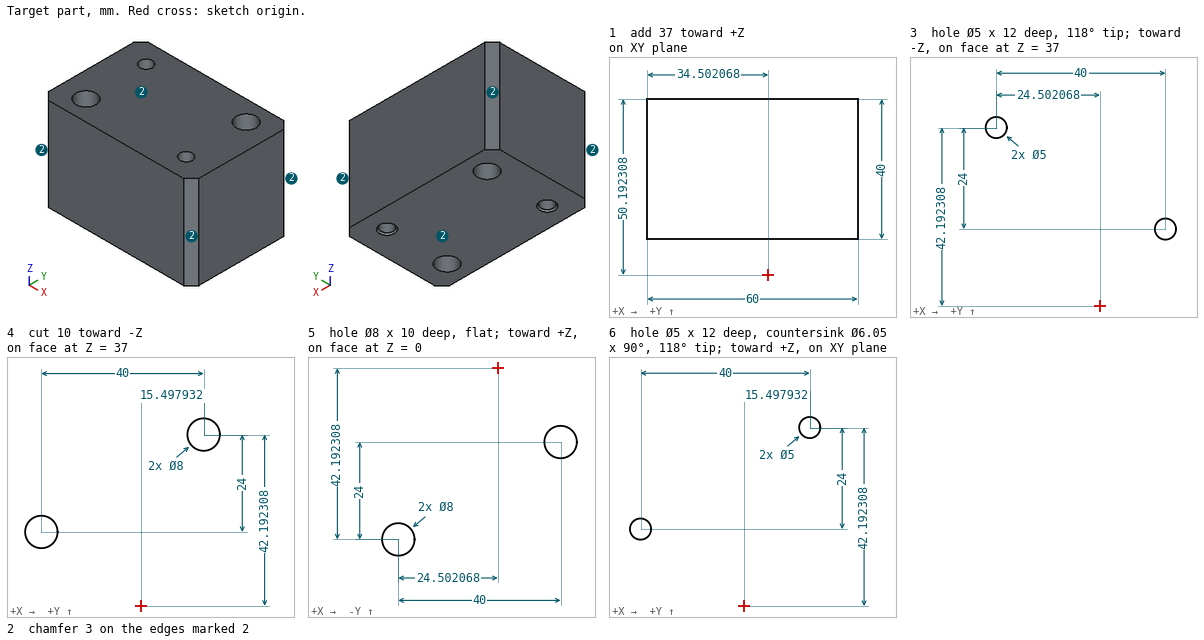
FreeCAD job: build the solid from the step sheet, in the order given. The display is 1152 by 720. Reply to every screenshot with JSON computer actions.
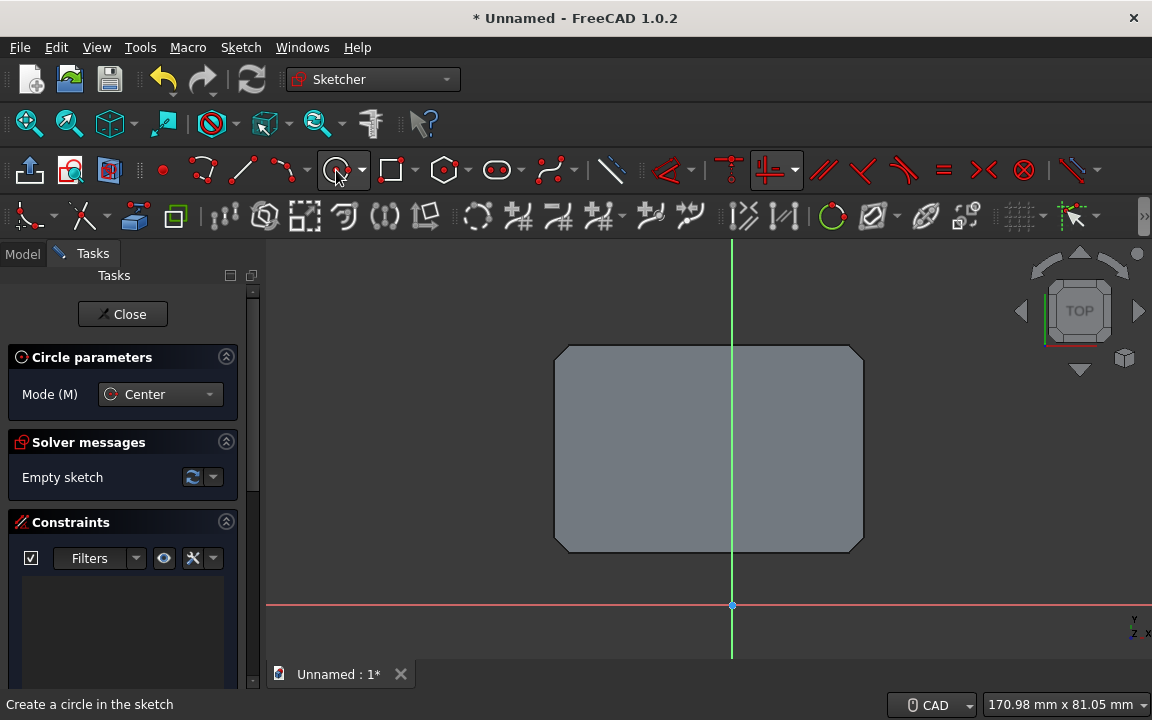
{"action": "scroll", "coordinate": [605, 387], "scroll_direction": "up", "scroll_amount": 3}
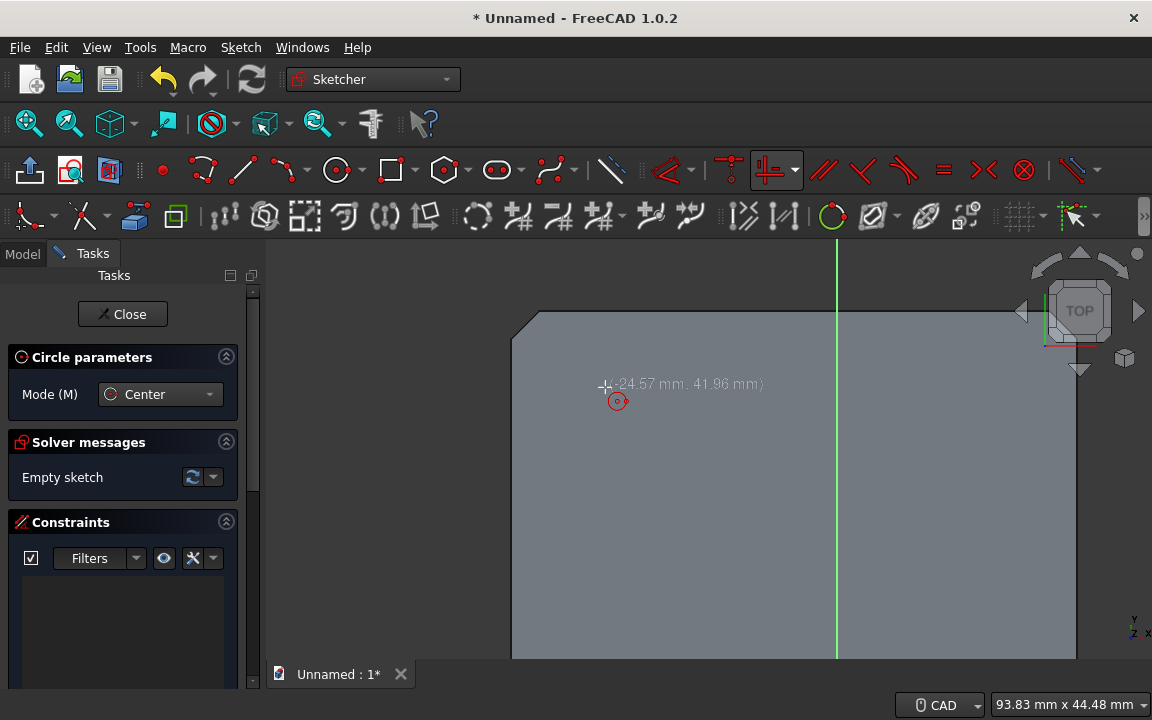
{"action": "left_click", "coordinate": [605, 386]}
{"action": "mouse_move", "coordinate": [622, 370]}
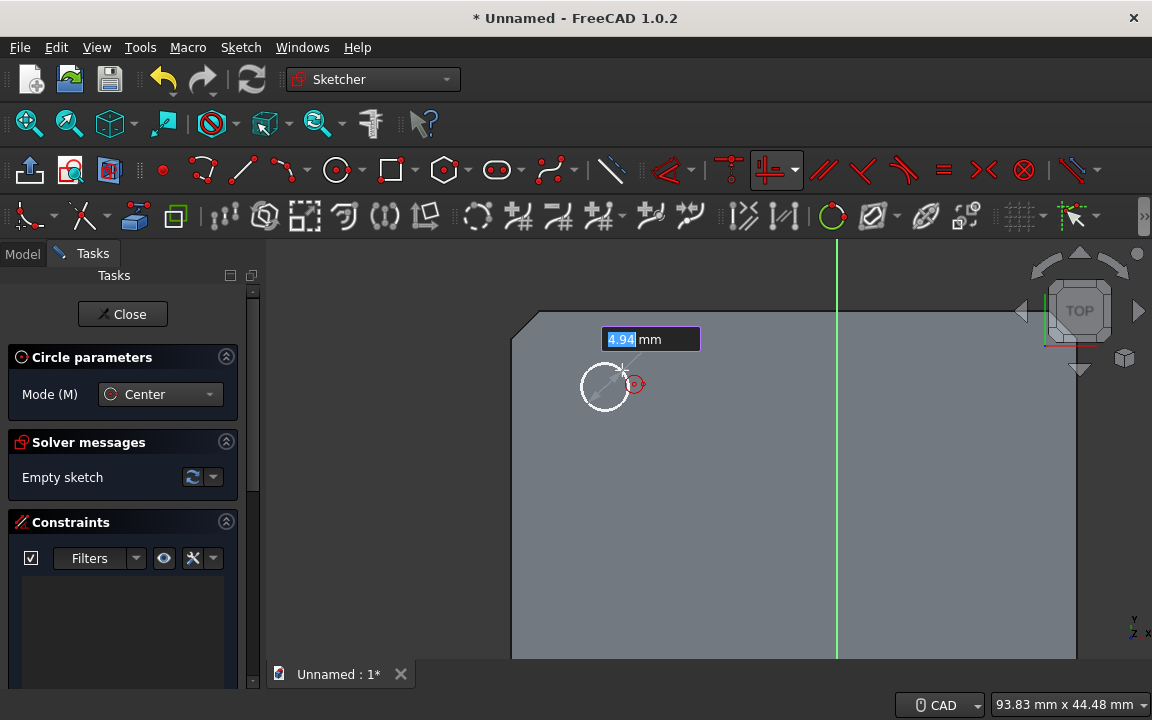
{"action": "type", "text": "5"}
{"action": "key", "text": "Return"}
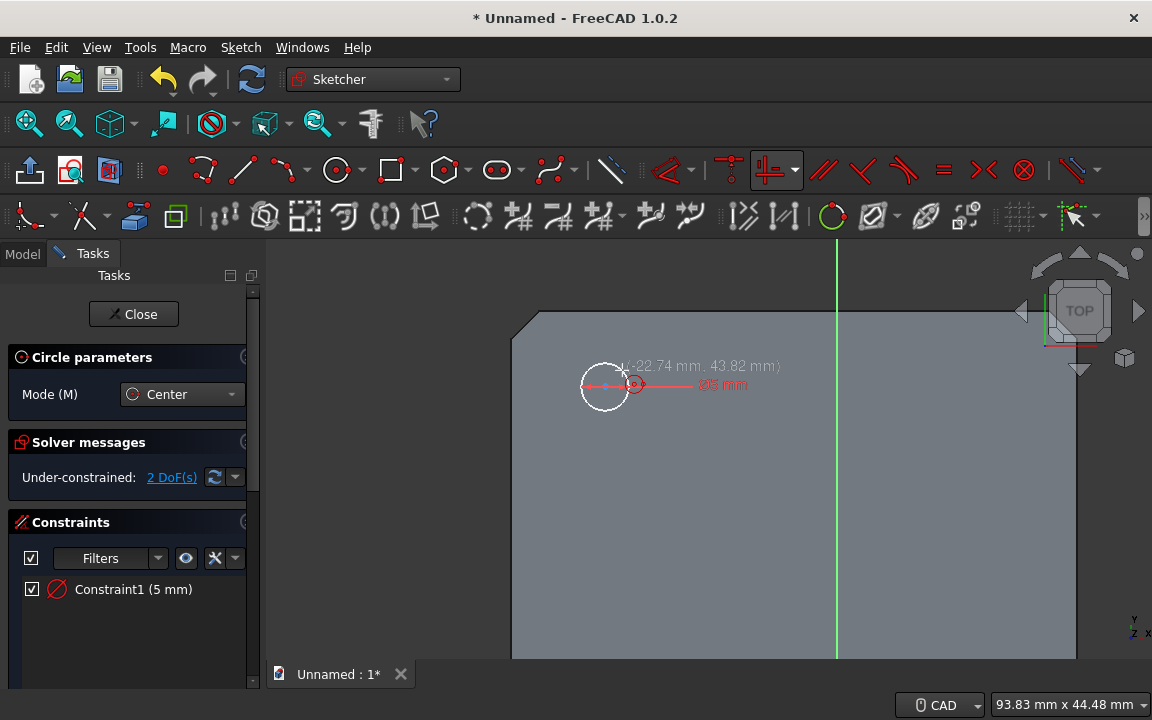
{"action": "left_click", "coordinate": [983, 613]}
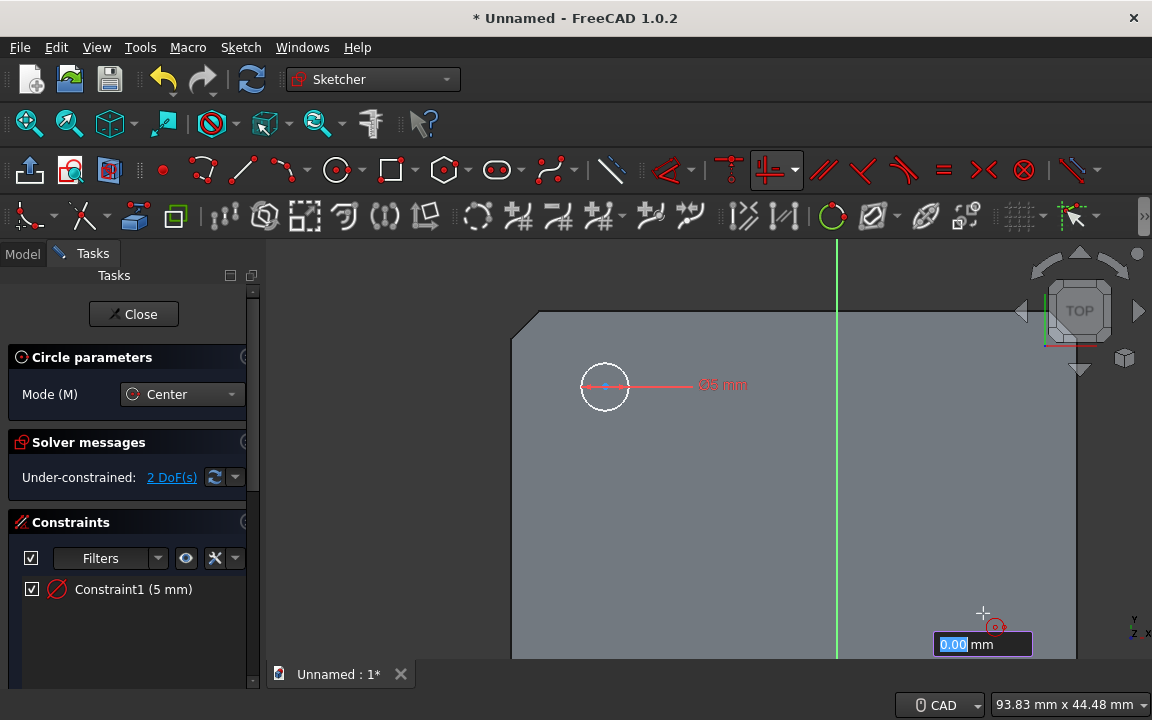
{"action": "scroll", "coordinate": [454, 297], "scroll_direction": "down", "scroll_amount": 3}
{"action": "mouse_move", "coordinate": [754, 461]}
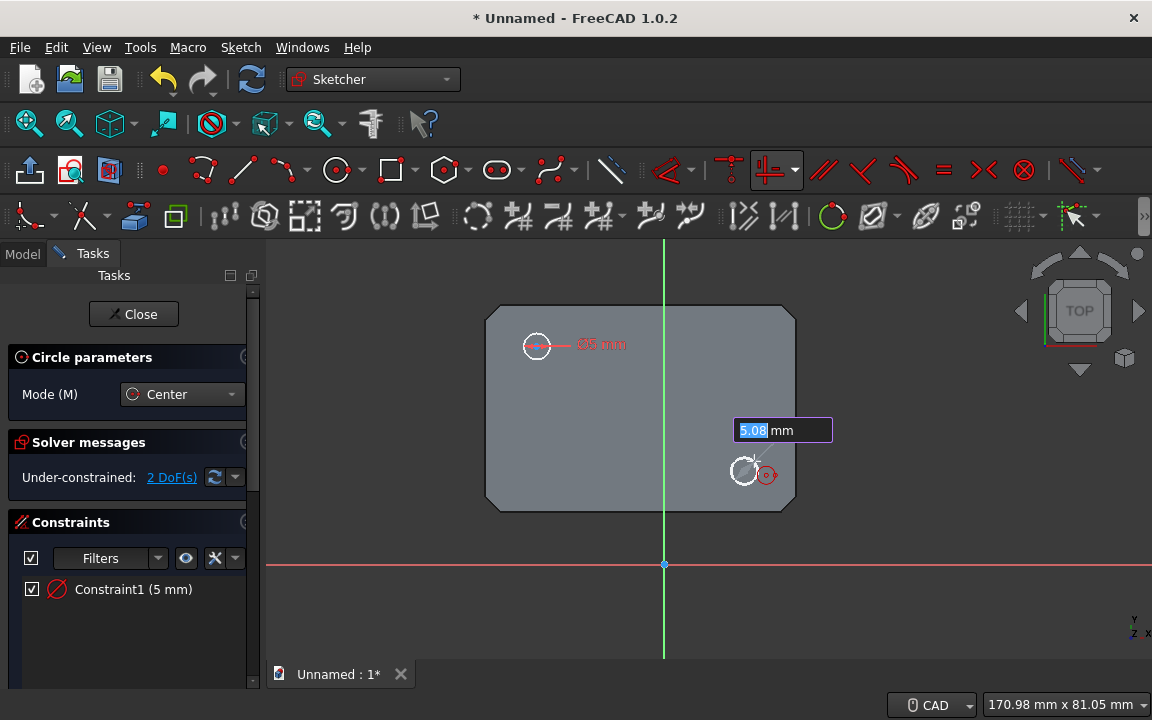
{"action": "type", "text": "5"}
{"action": "key", "text": "Return"}
{"action": "key", "text": "Escape"}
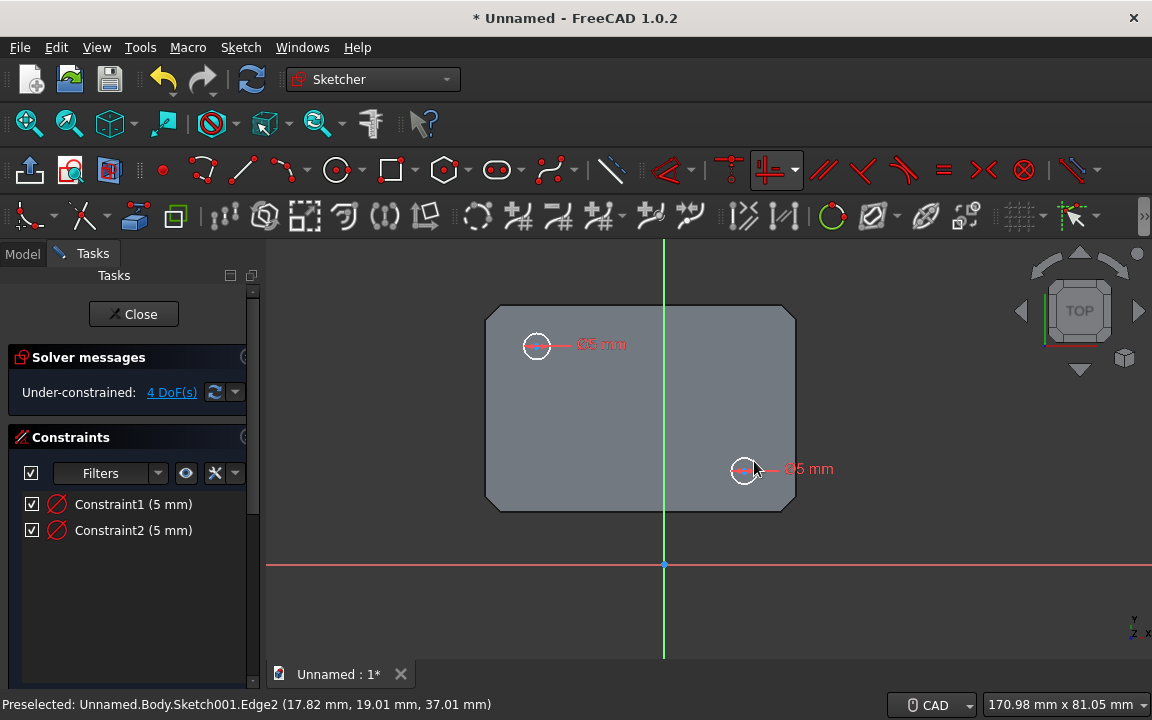
{"action": "left_click", "coordinate": [666, 170]}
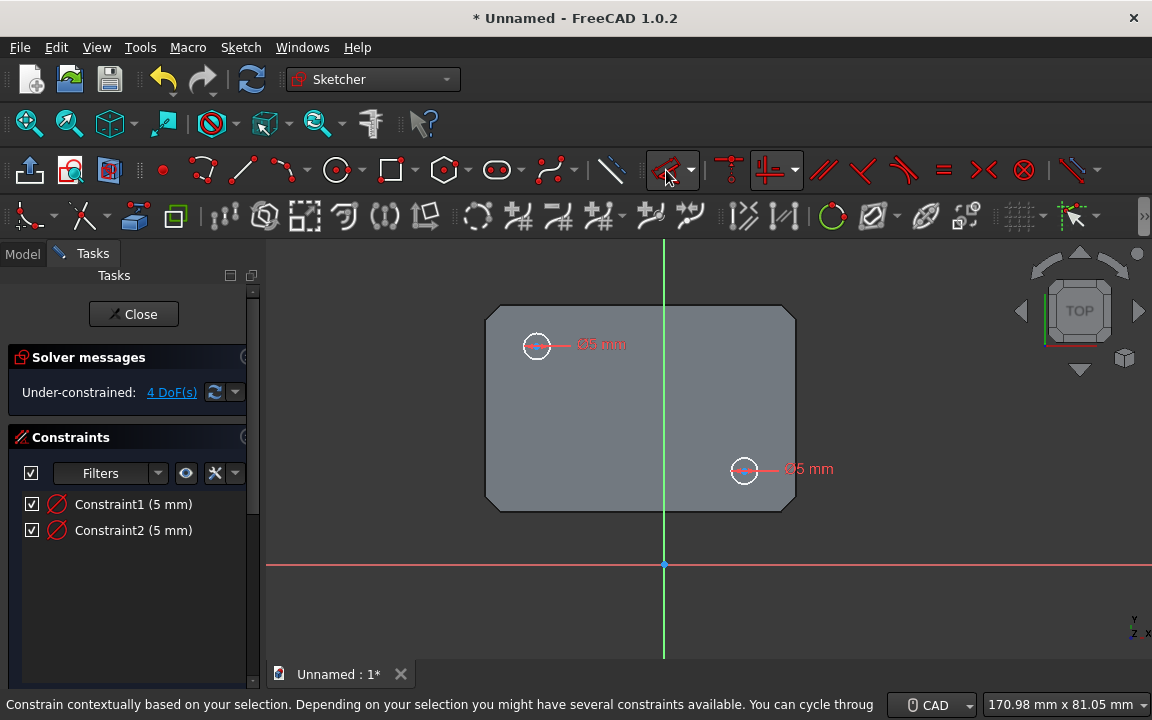
{"action": "left_click", "coordinate": [537, 346]}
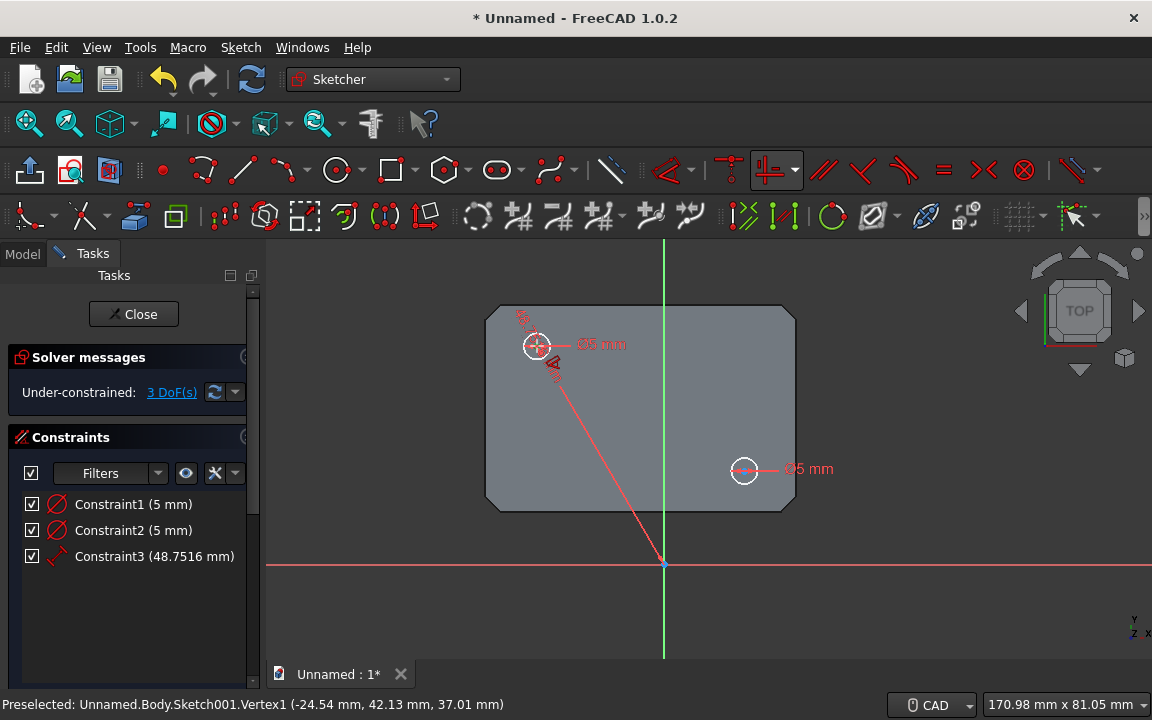
{"action": "left_click", "coordinate": [744, 471]}
{"action": "left_click", "coordinate": [641, 312]}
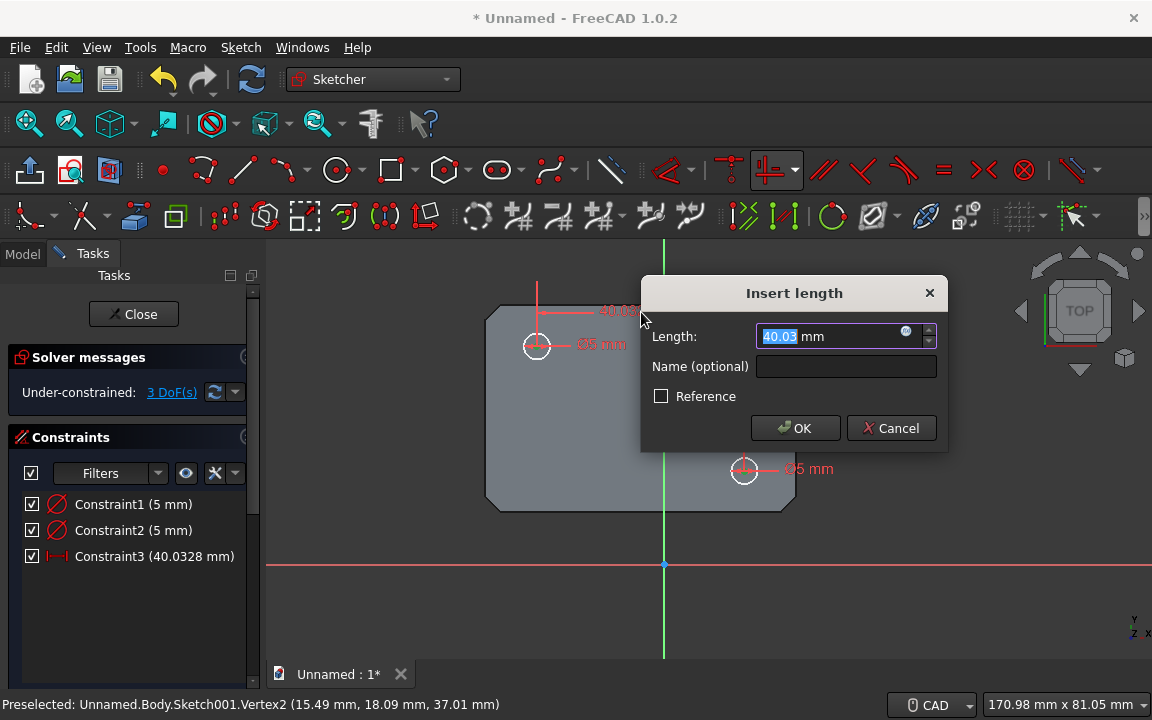
{"action": "type", "text": "40"}
{"action": "key", "text": "Return"}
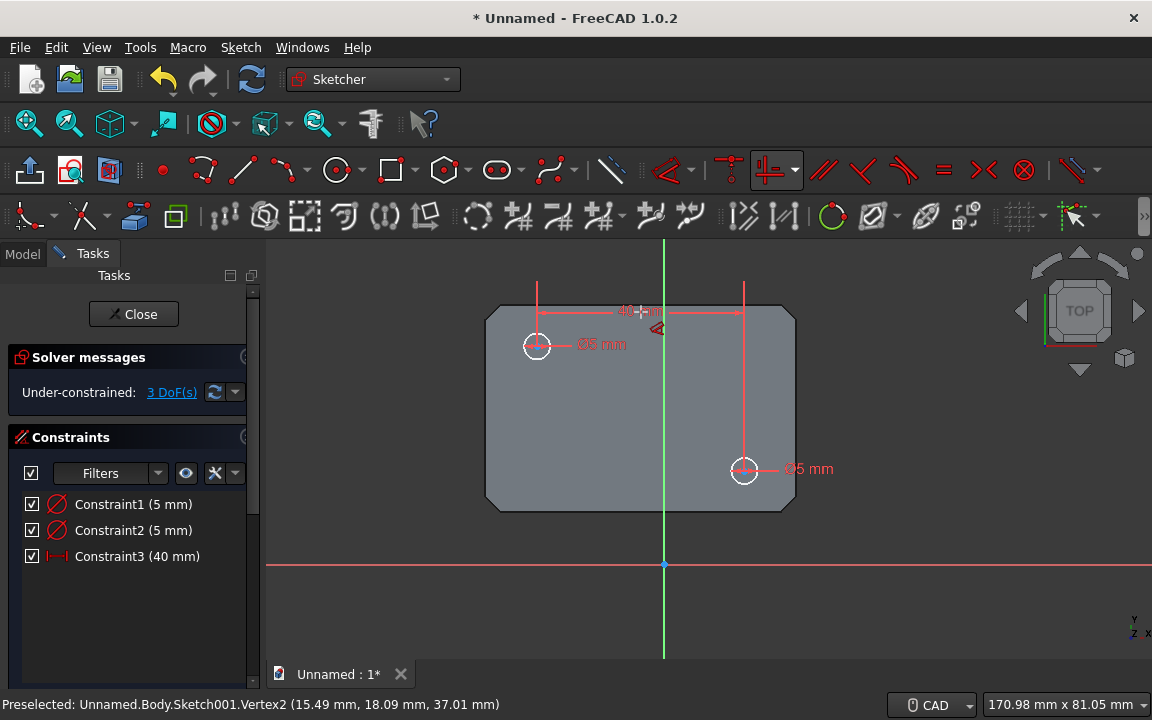
{"action": "left_click", "coordinate": [537, 346]}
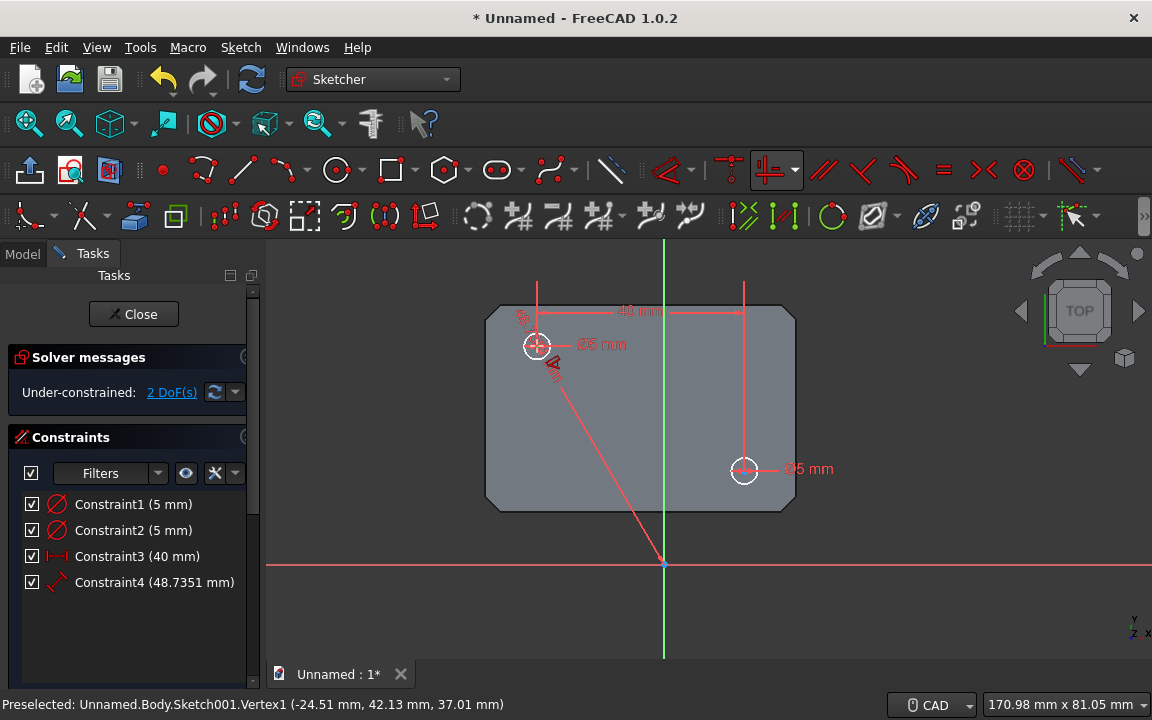
{"action": "left_click", "coordinate": [744, 471]}
{"action": "left_click", "coordinate": [503, 409]}